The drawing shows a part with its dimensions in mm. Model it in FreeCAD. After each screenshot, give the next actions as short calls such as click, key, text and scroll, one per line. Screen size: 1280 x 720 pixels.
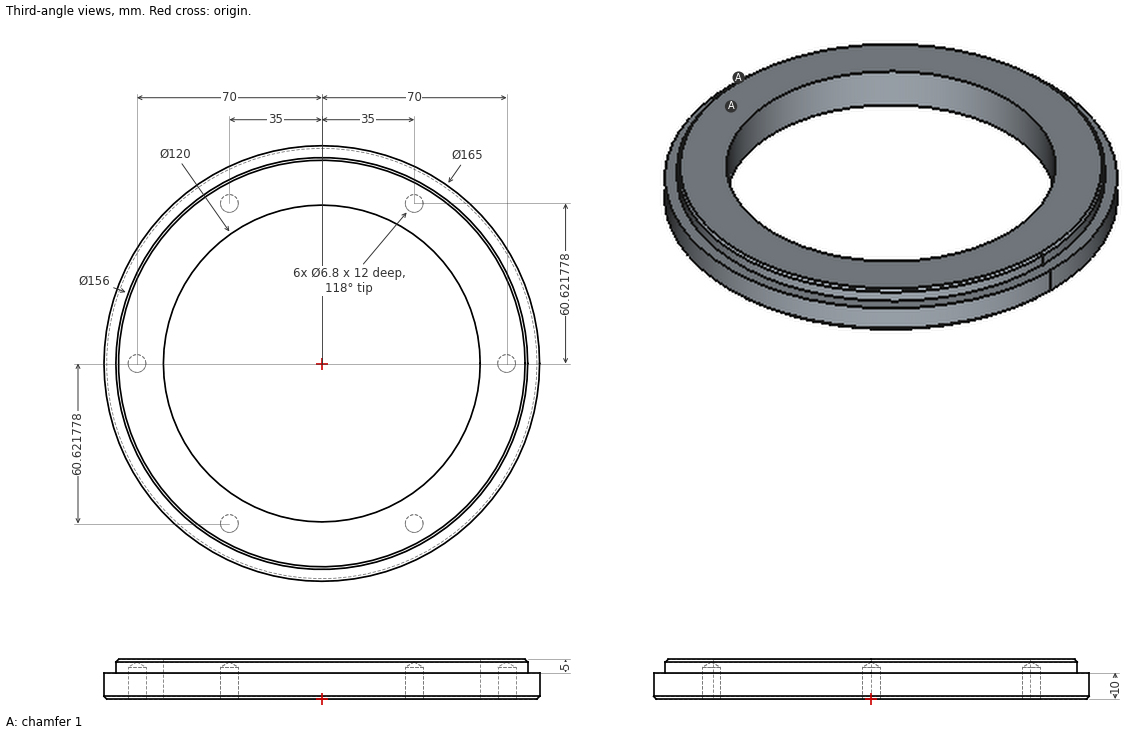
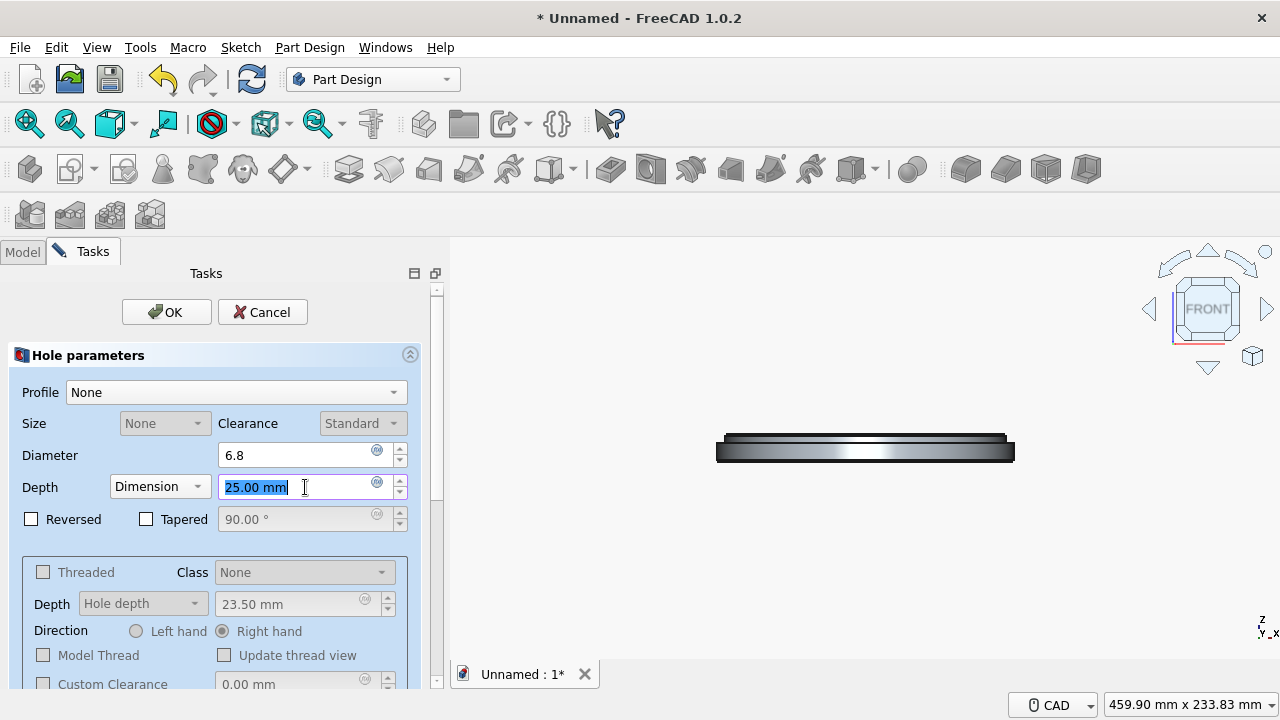
text(12)
key(Tab)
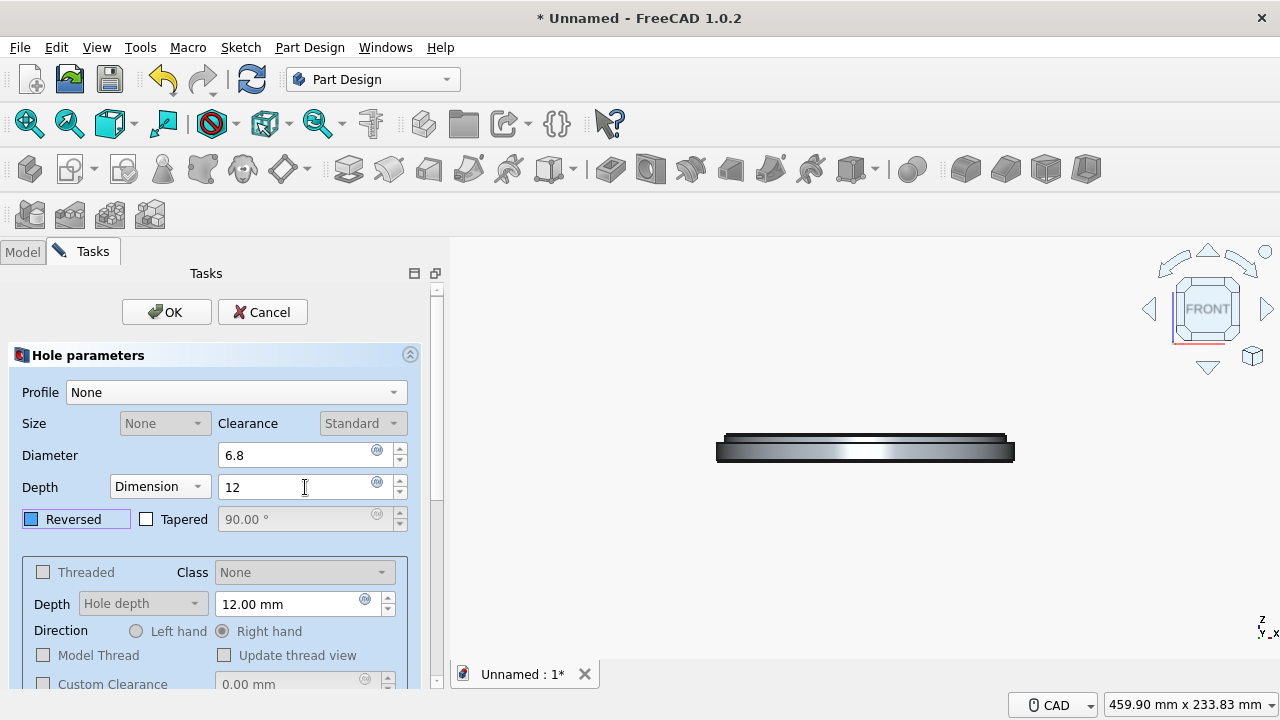
click(30, 519)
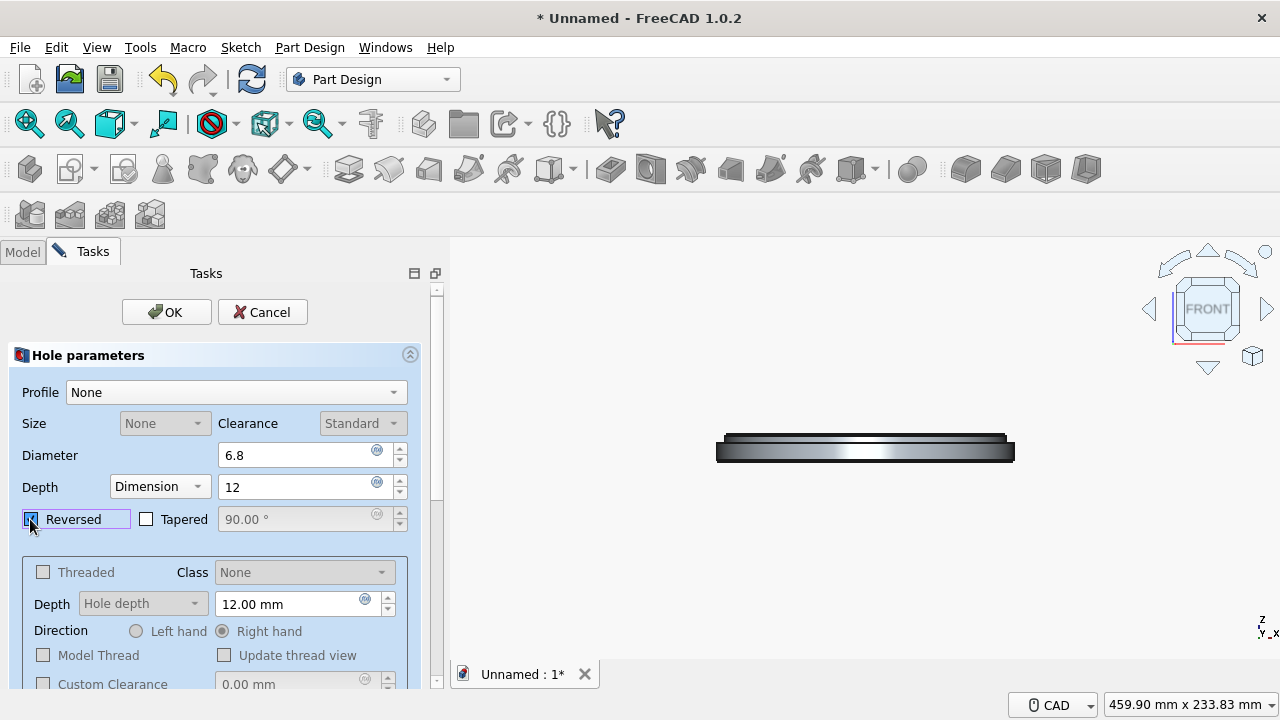
click(167, 312)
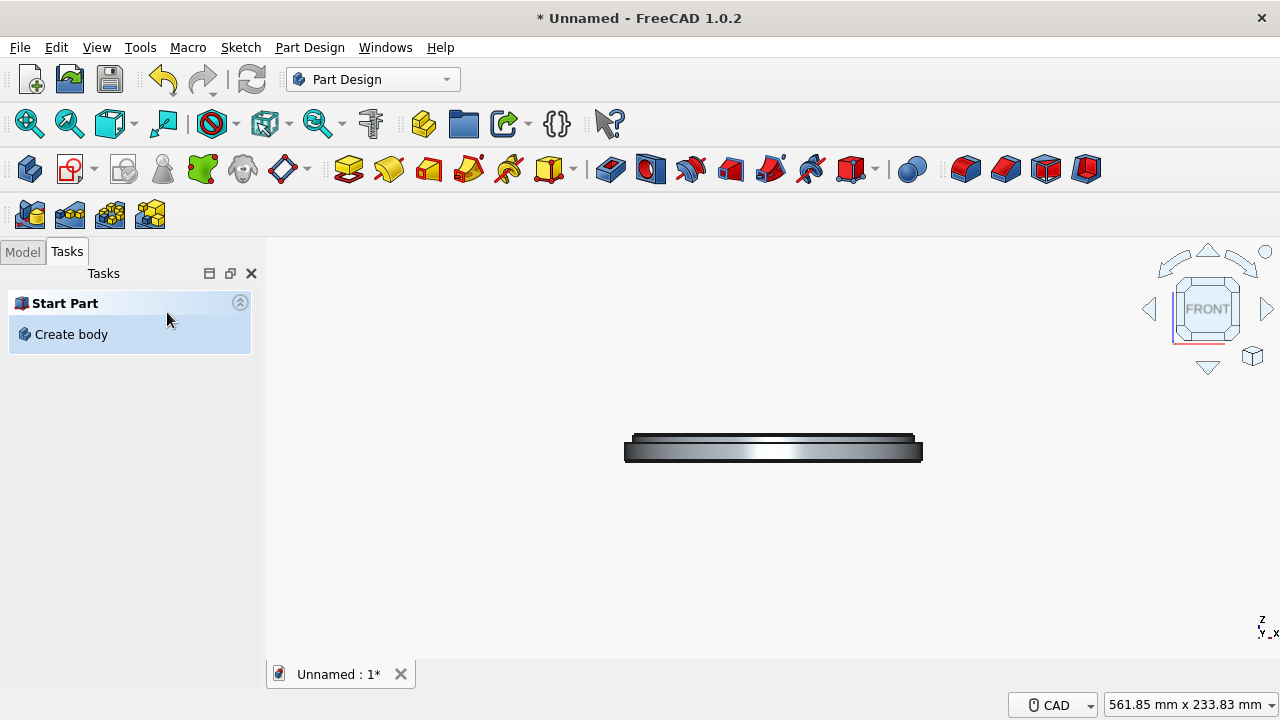
key(0)